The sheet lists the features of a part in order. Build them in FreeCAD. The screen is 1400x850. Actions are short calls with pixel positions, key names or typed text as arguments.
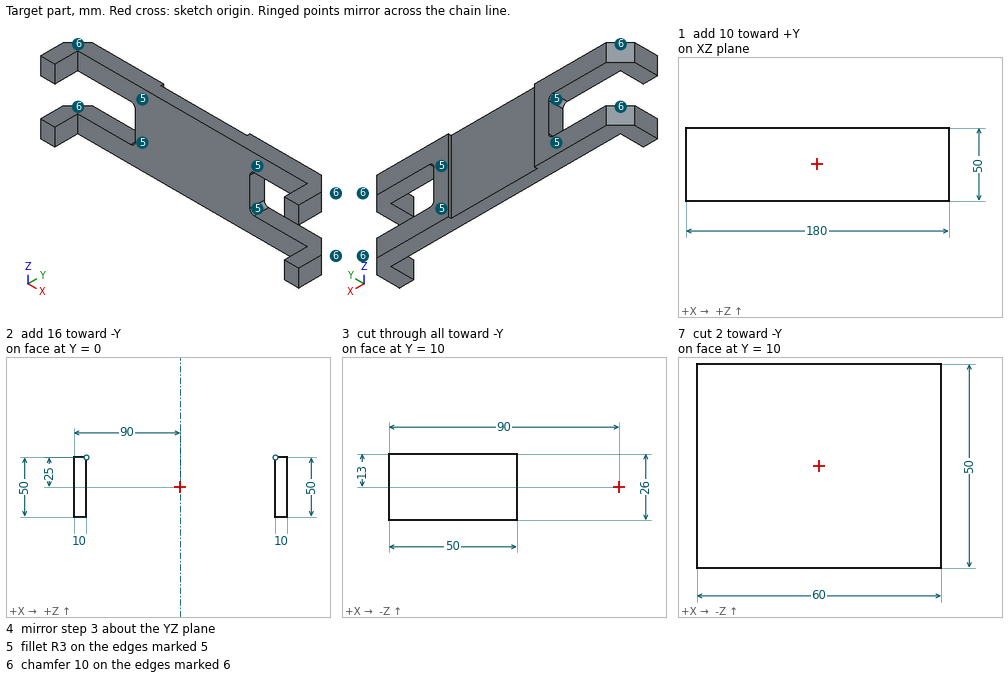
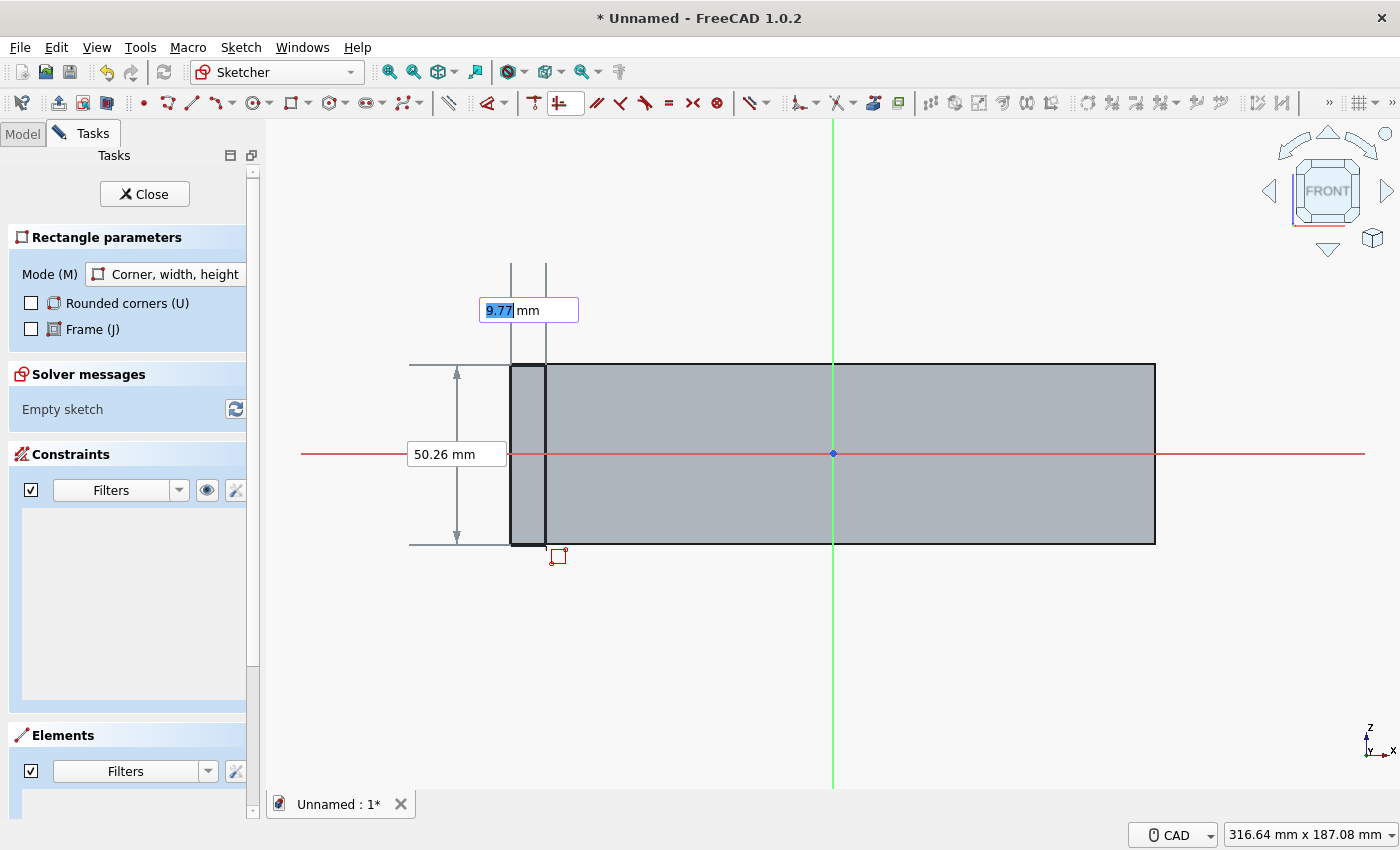
text(10)
key(Tab)
text(50)
key(Return)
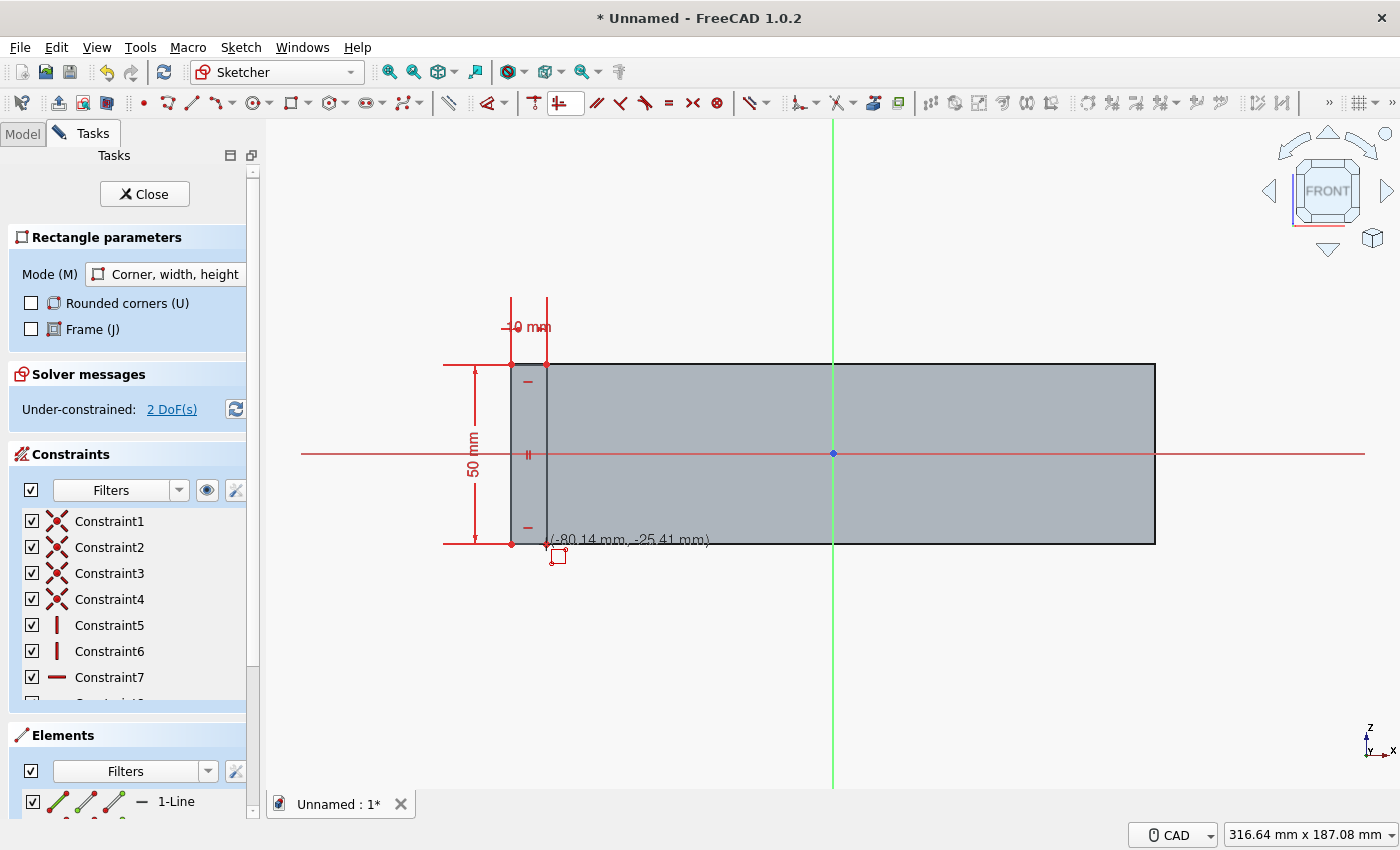
click(1120, 364)
move(1155, 544)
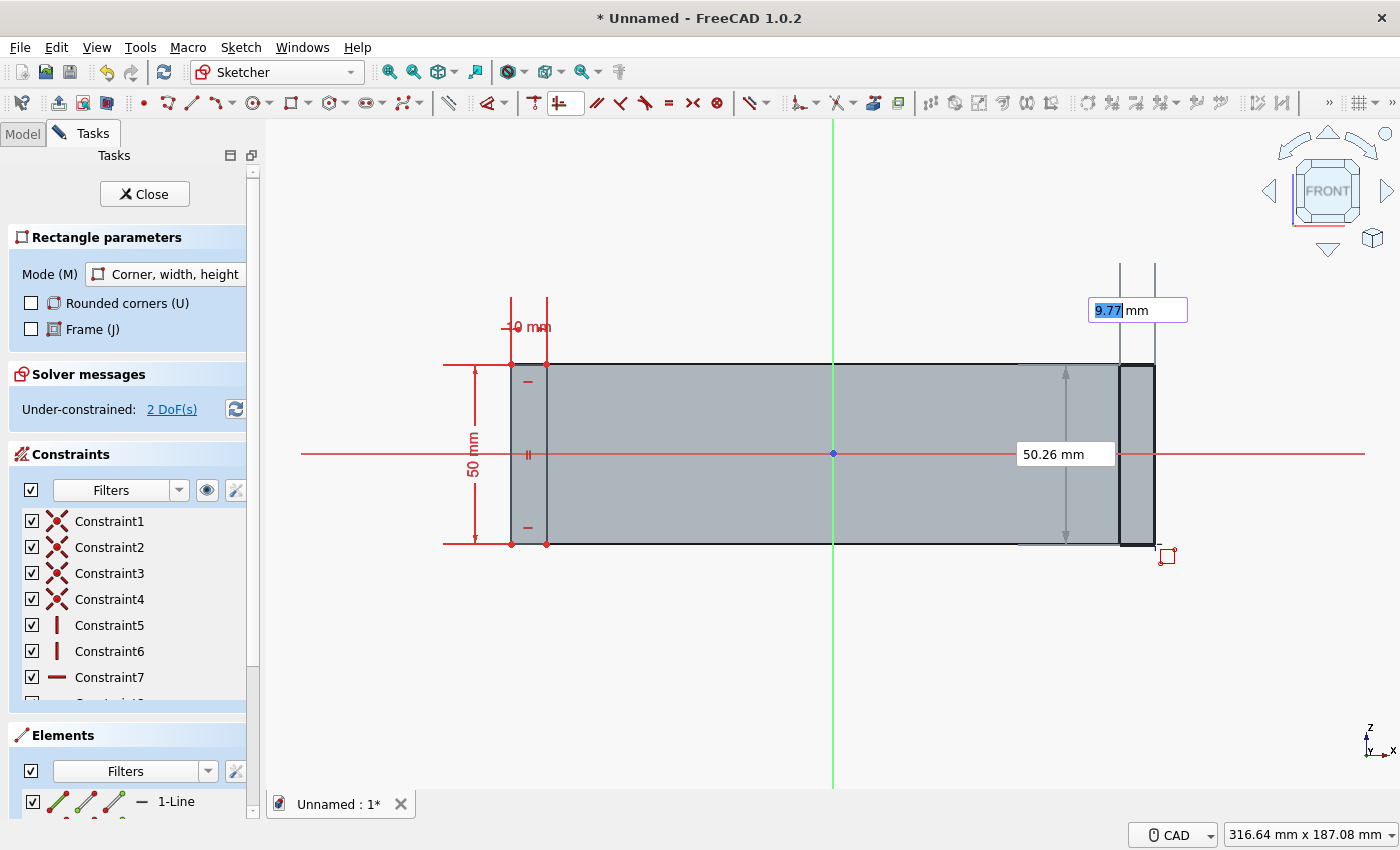
text(10)
key(Tab)
text(50)
key(Return)
key(Escape)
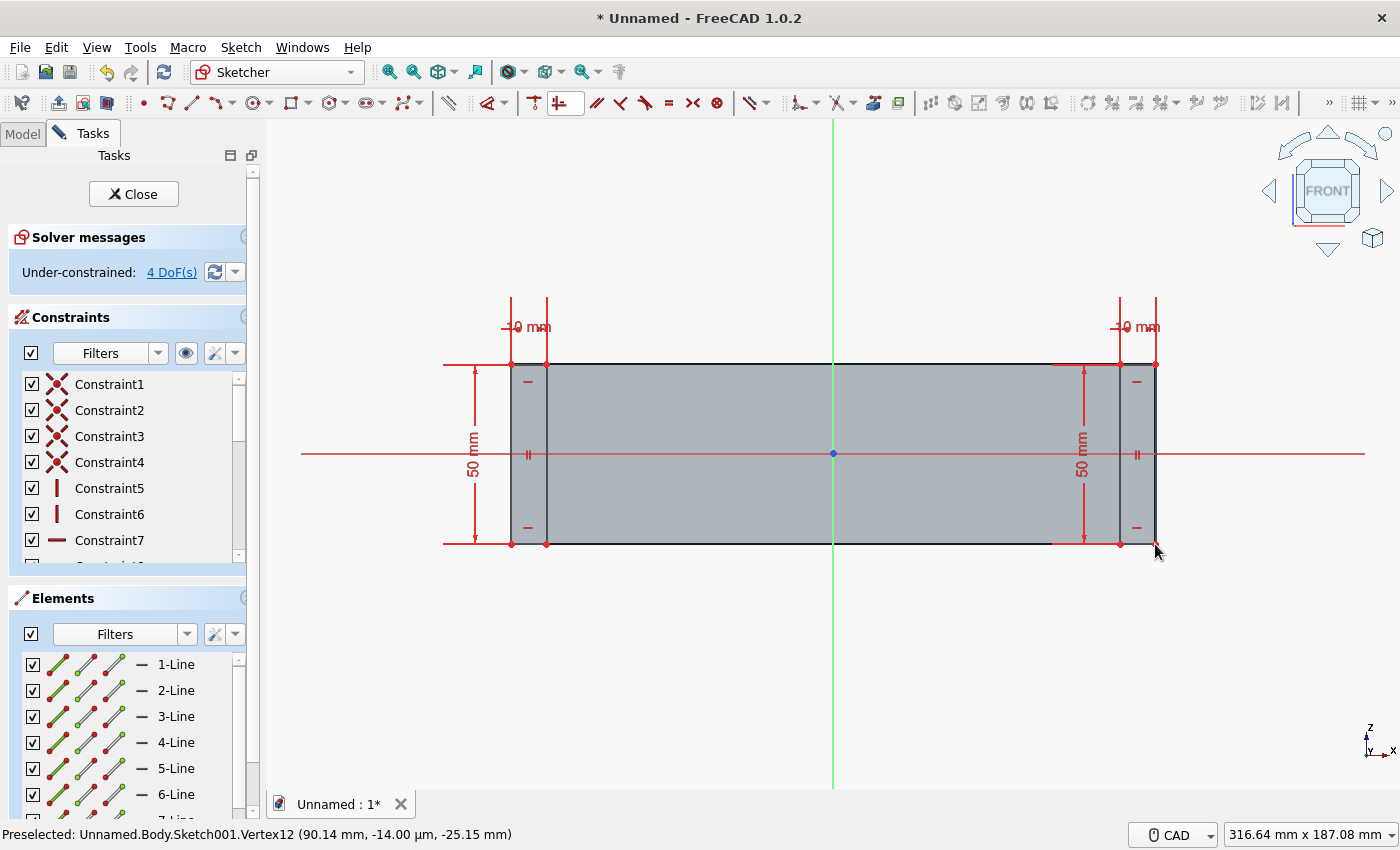
click(547, 365)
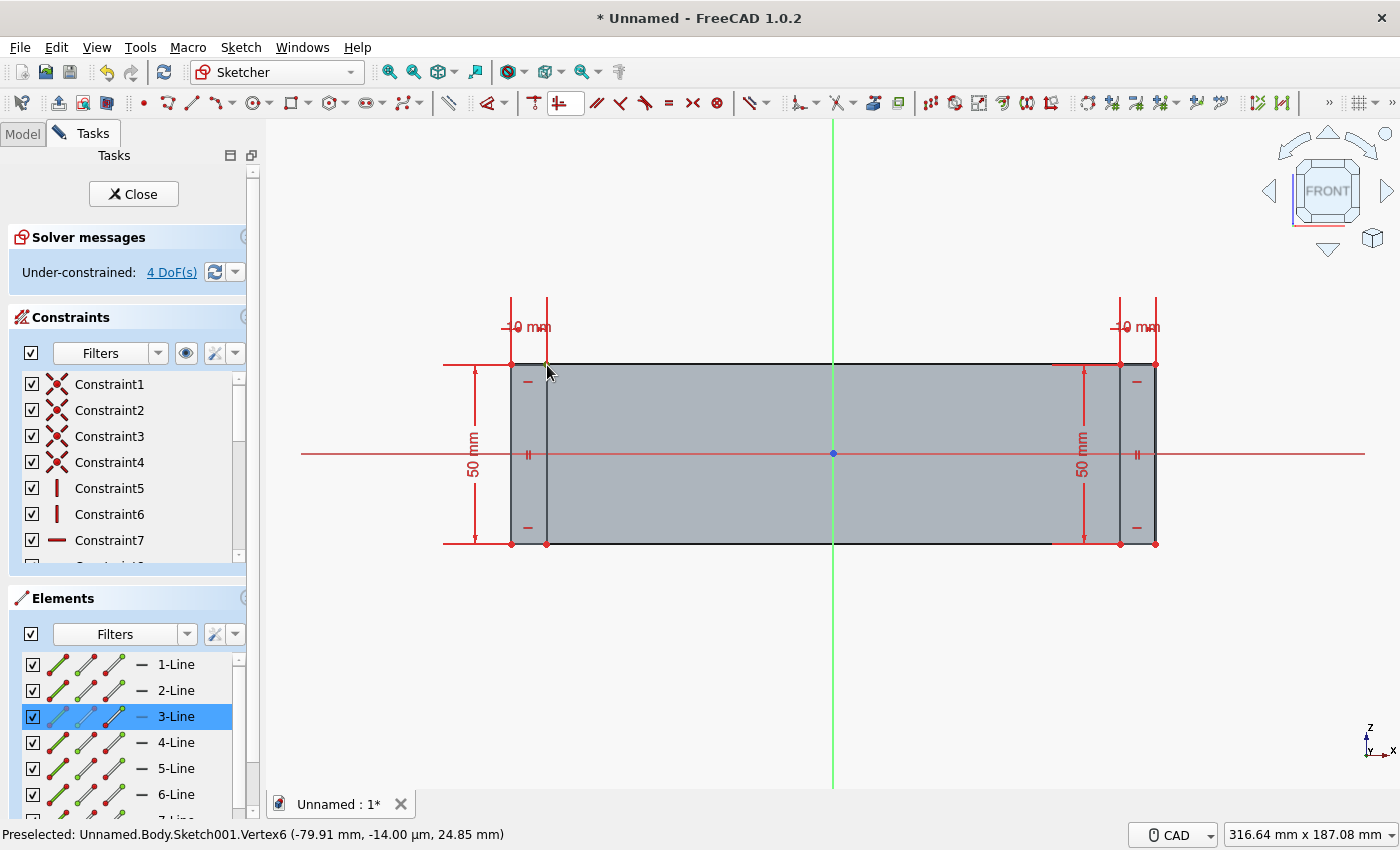
click(1120, 365)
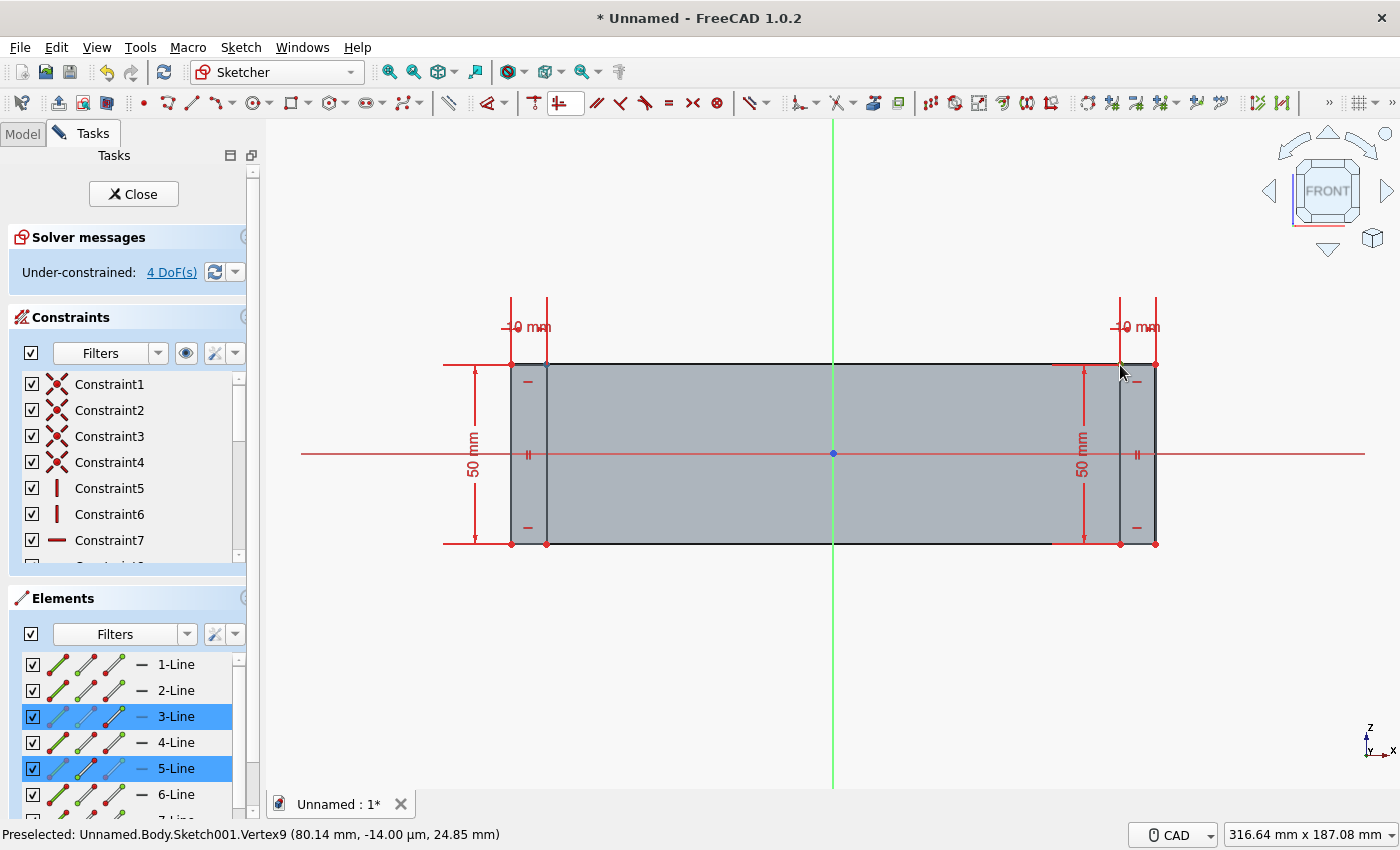
click(833, 717)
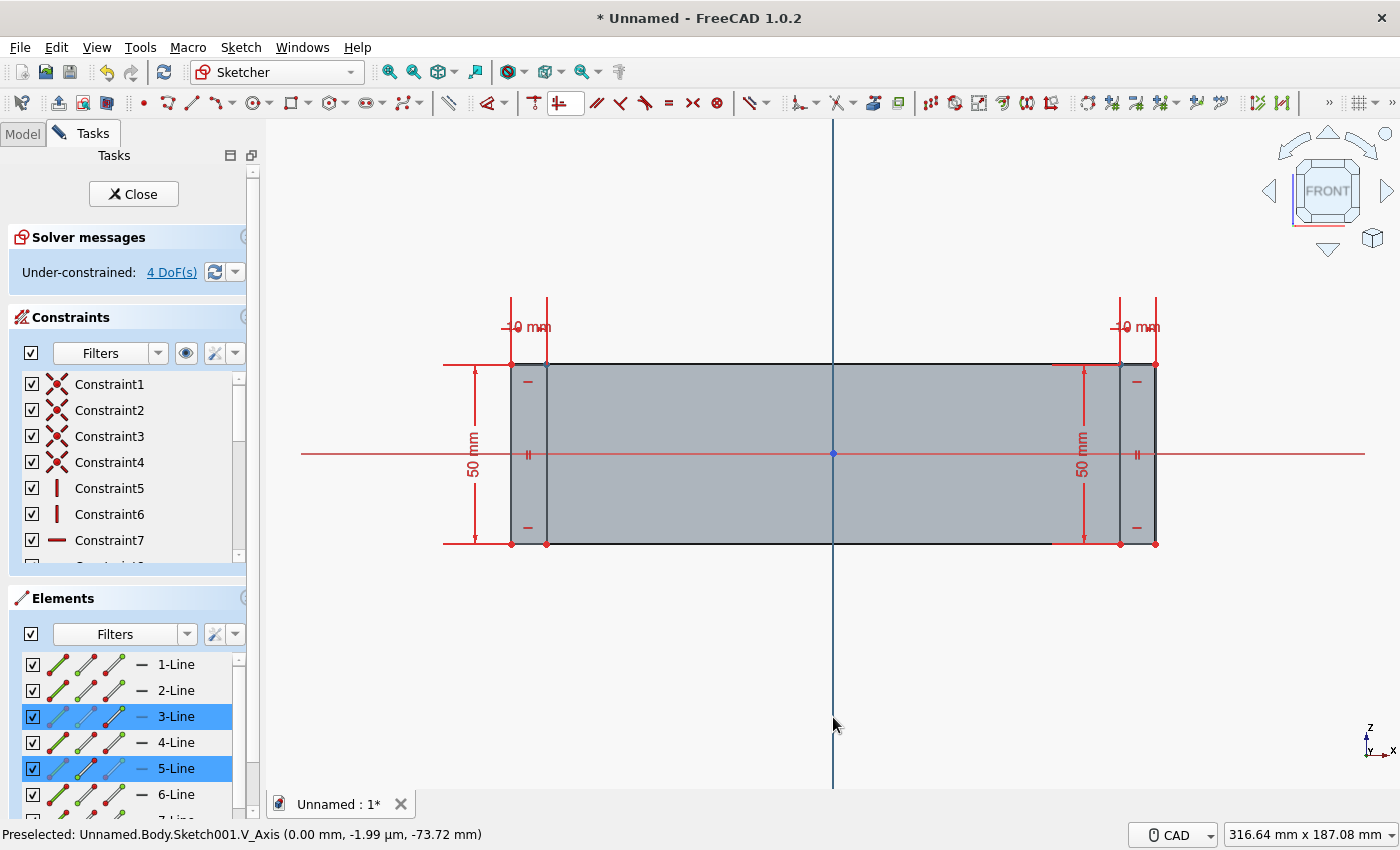
key(s)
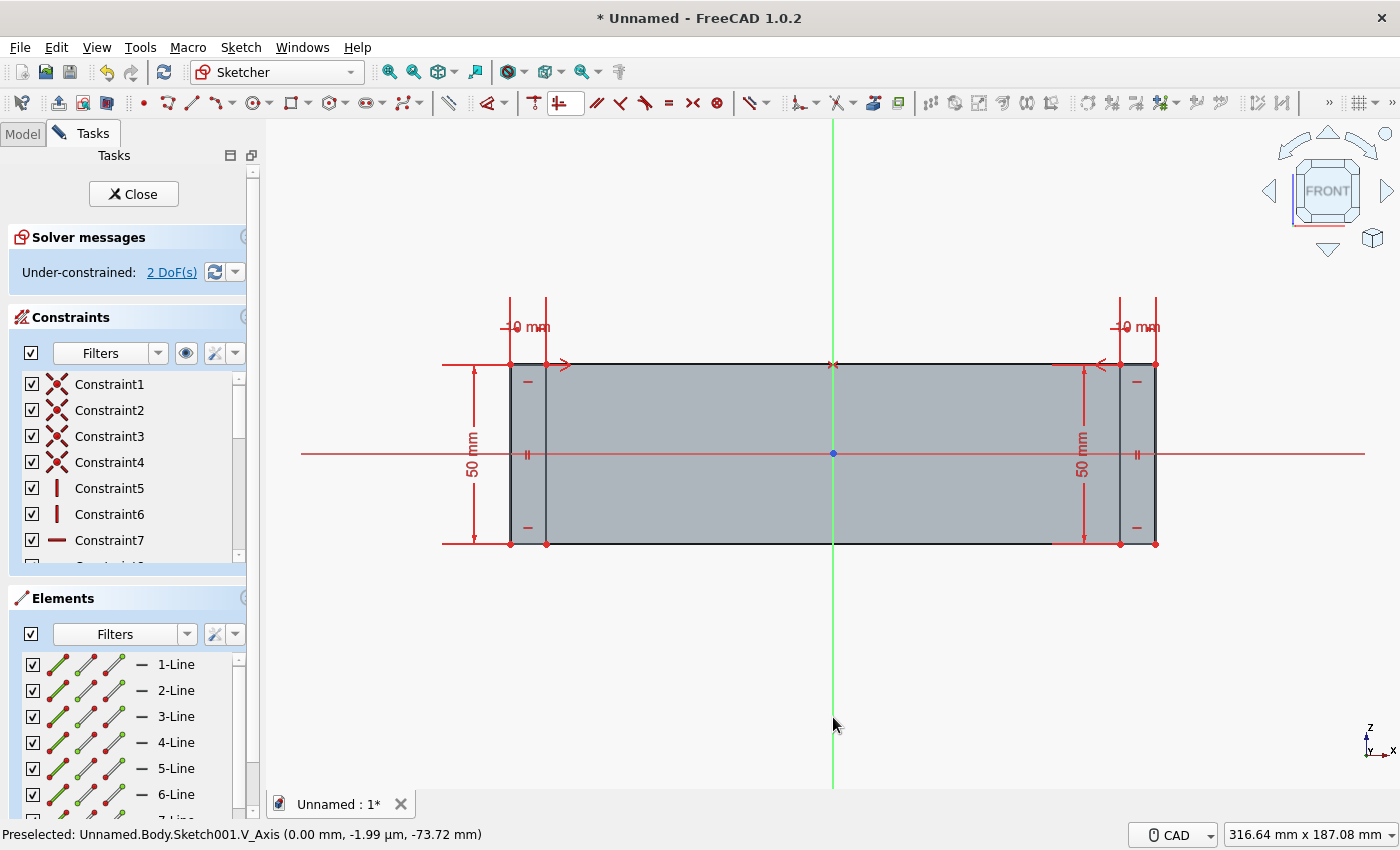
click(510, 365)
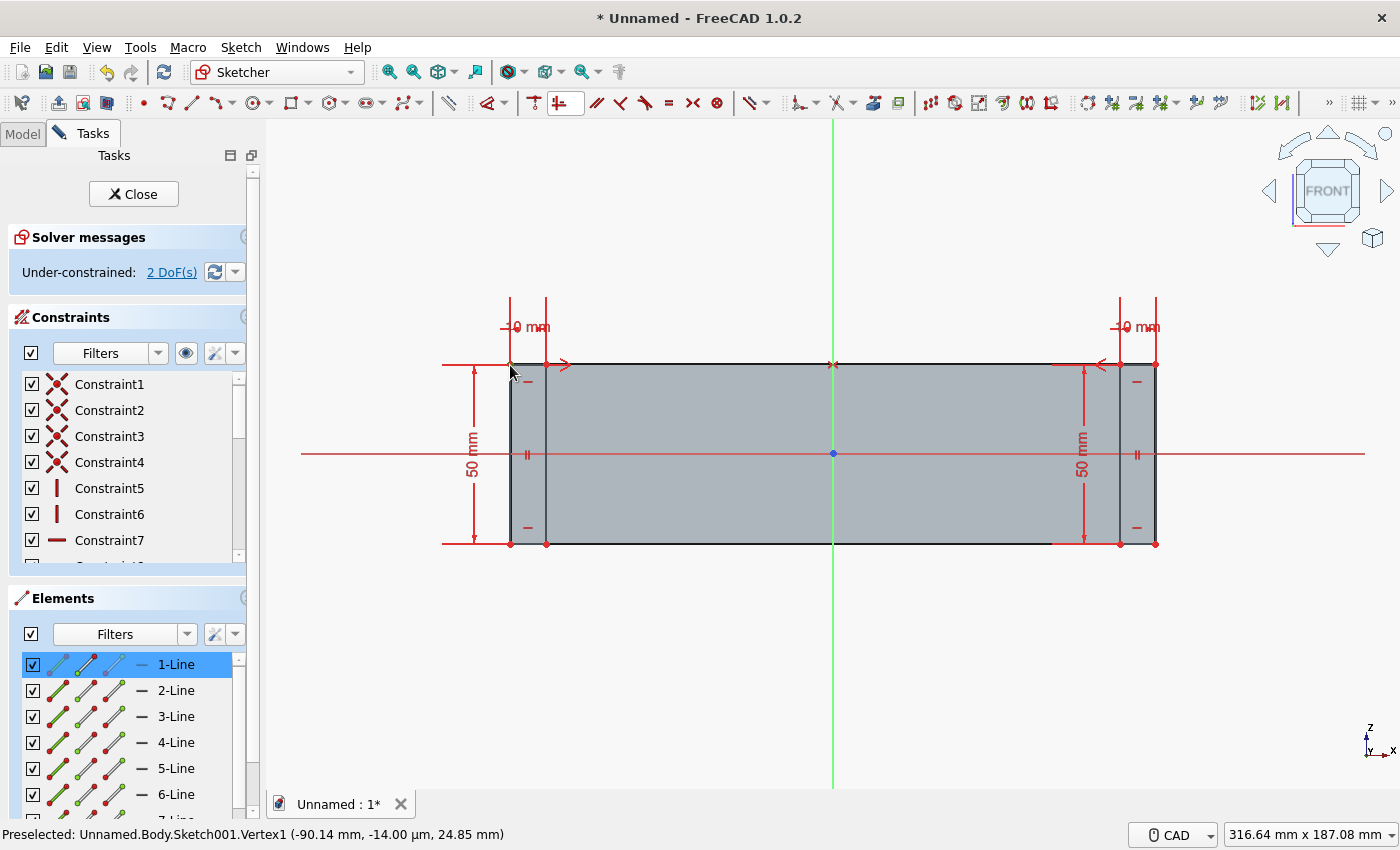
key(l)